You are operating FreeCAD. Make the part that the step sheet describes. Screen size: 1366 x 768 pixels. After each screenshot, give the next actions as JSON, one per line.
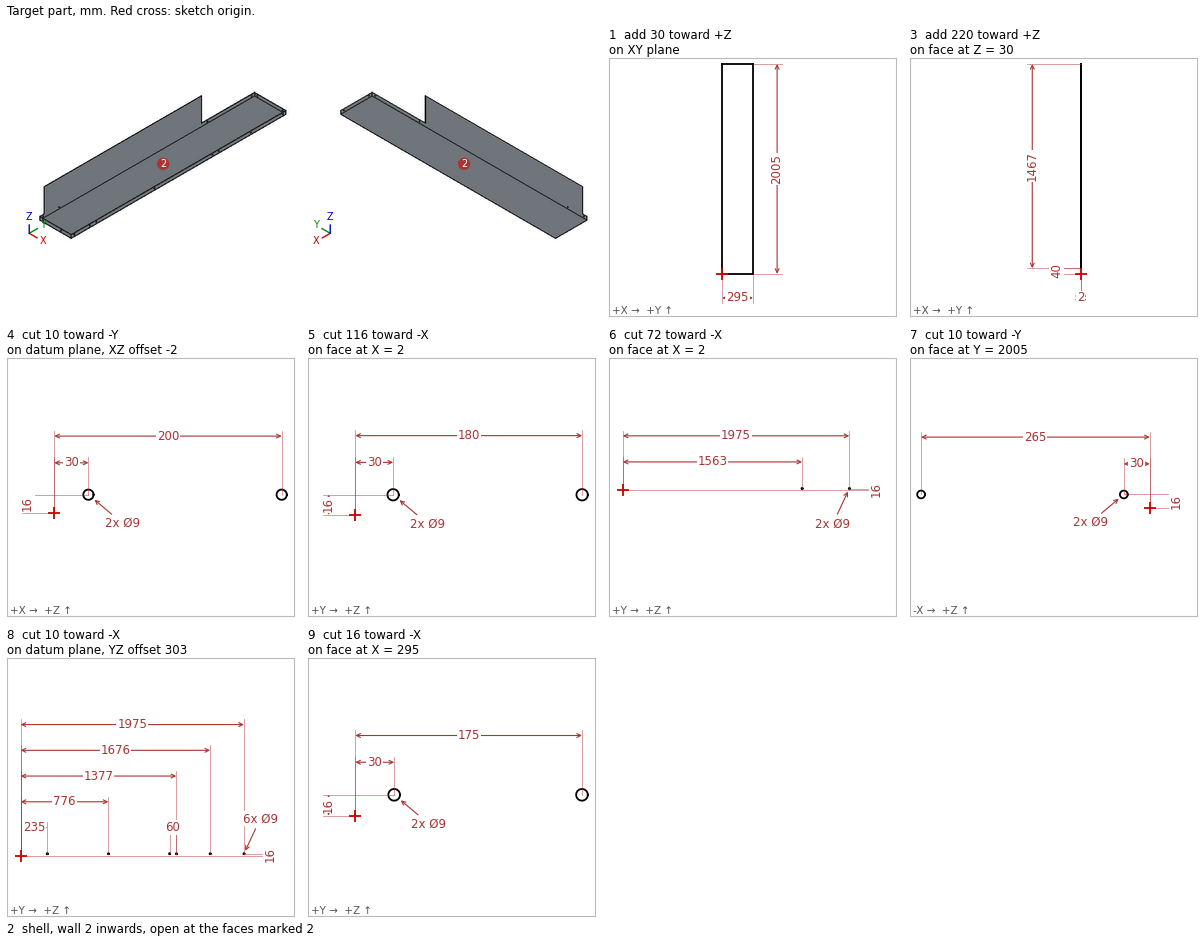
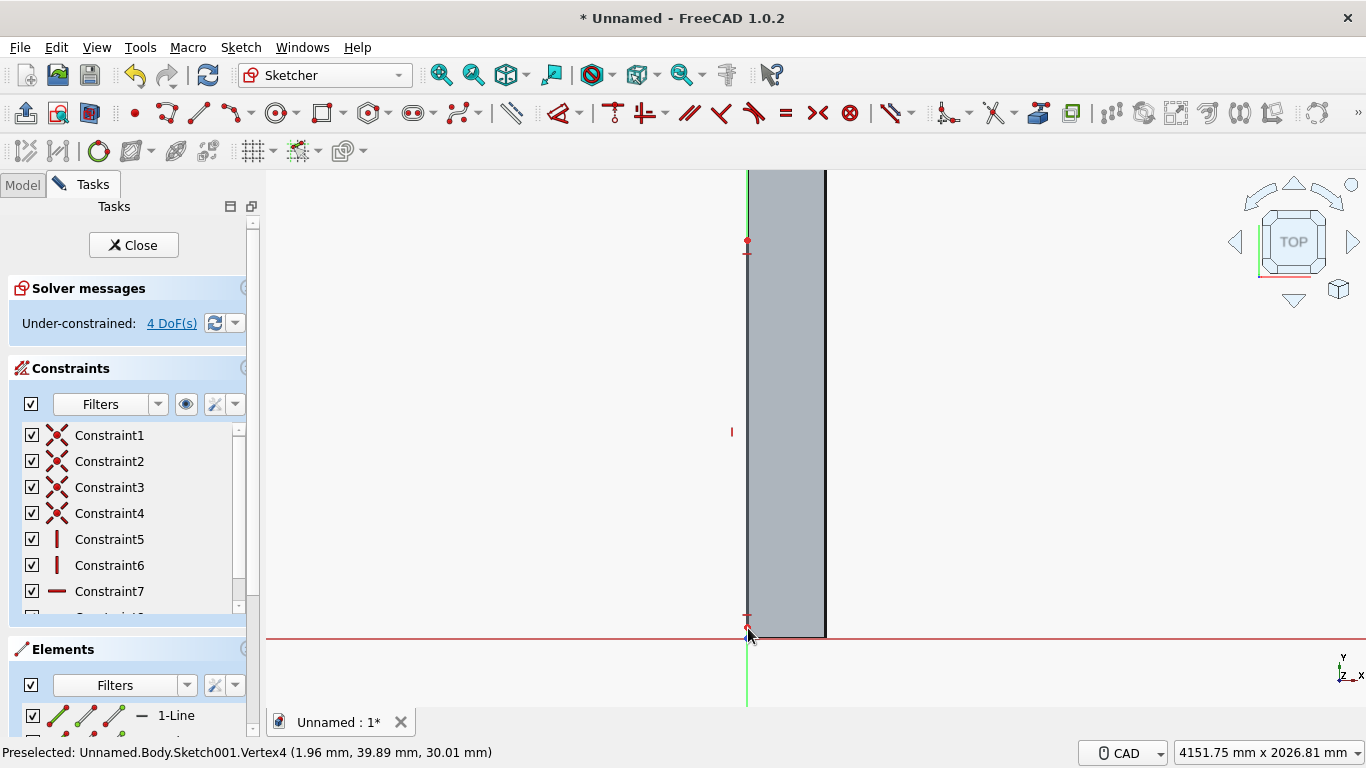
{"action": "scroll", "coordinate": [747, 240], "scroll_direction": "up", "scroll_amount": 13}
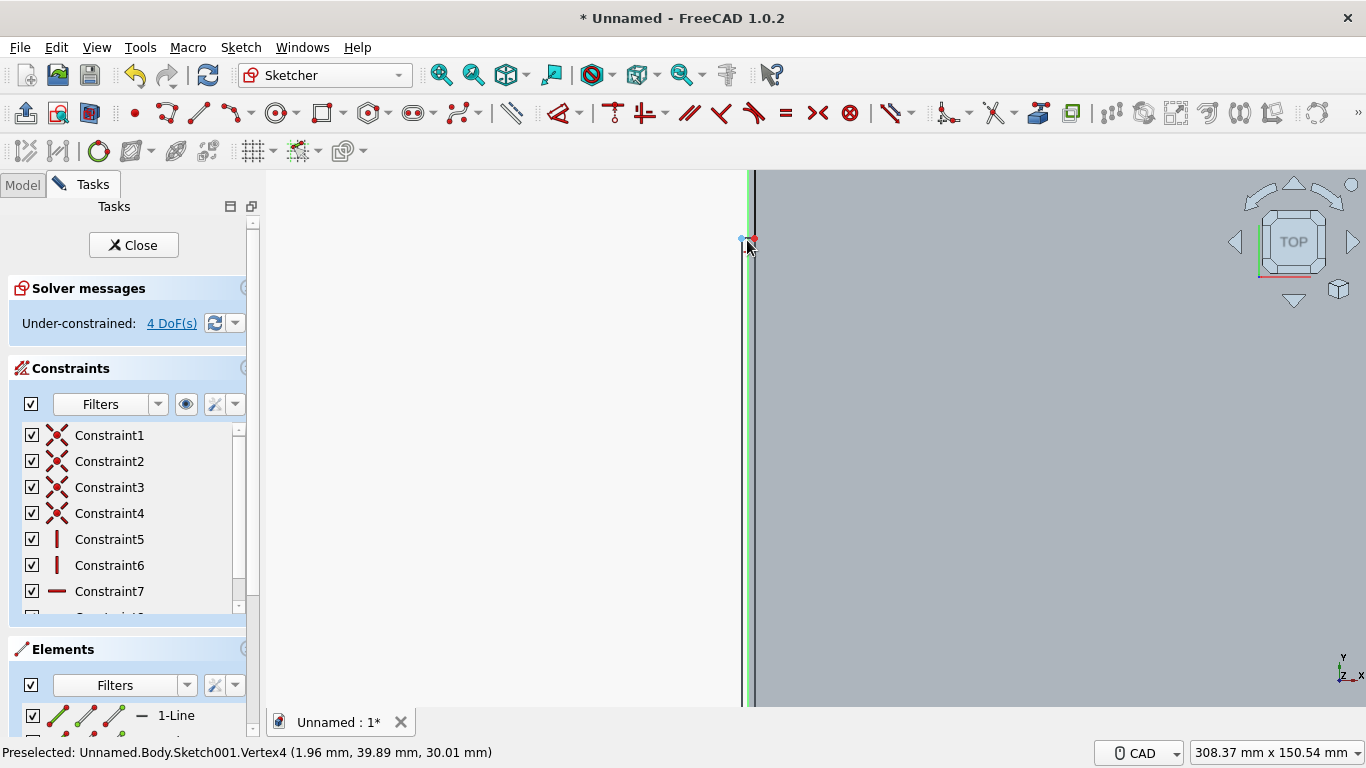
{"action": "left_click", "coordinate": [742, 238]}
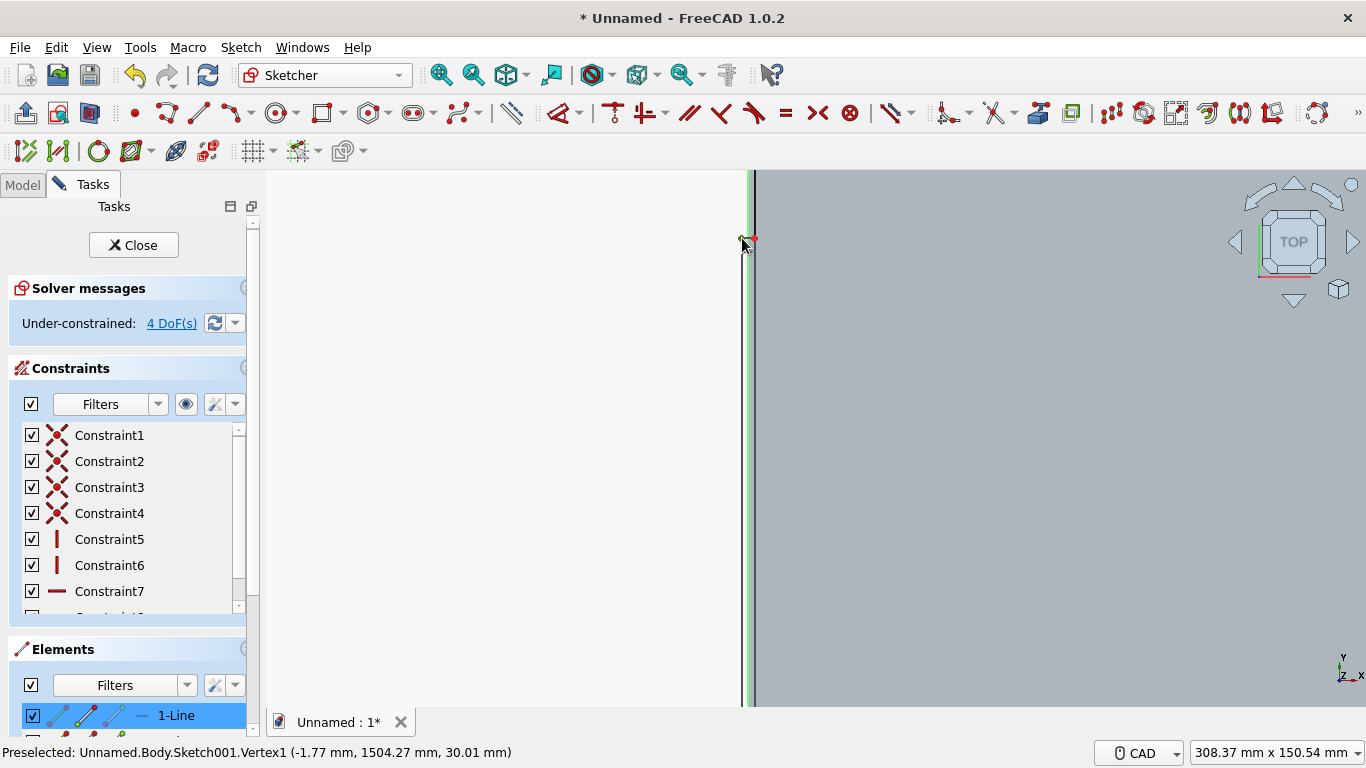
{"action": "left_click", "coordinate": [748, 645]}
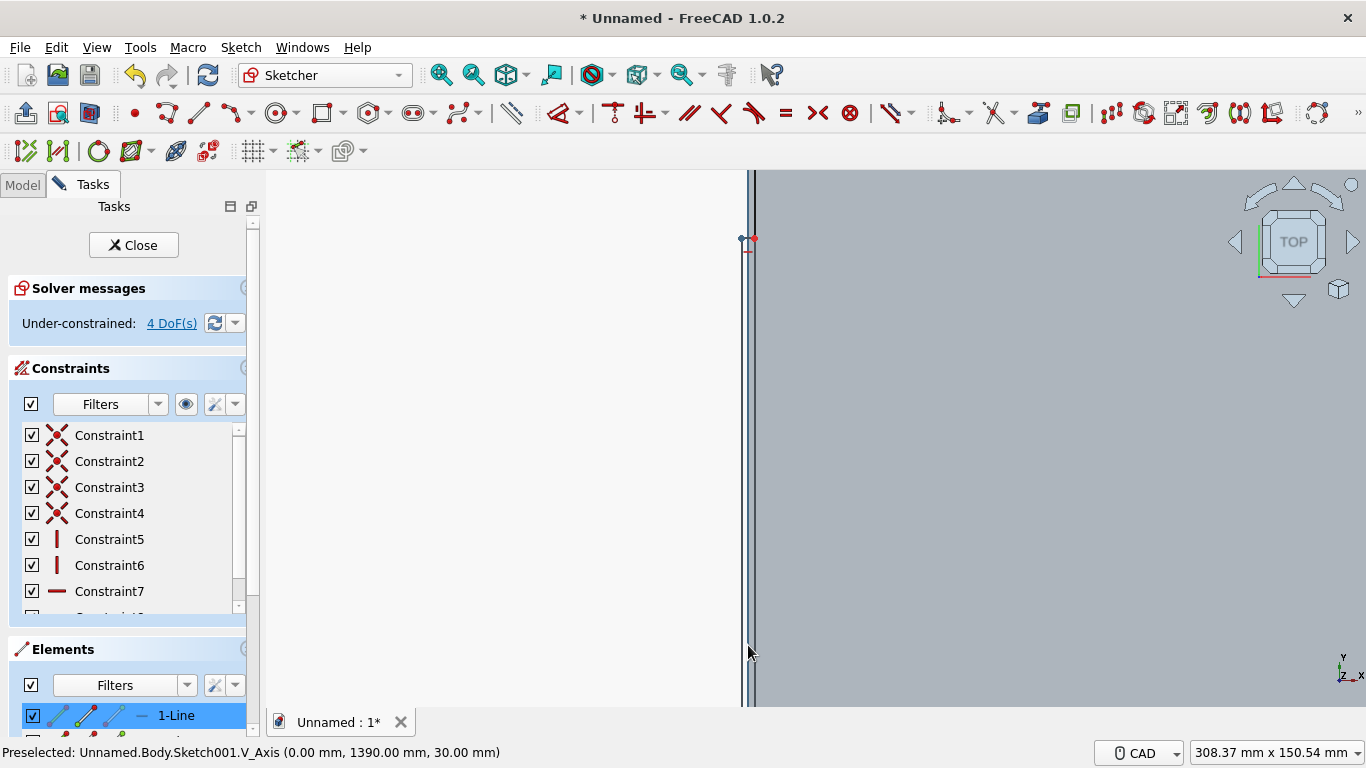
{"action": "left_click", "coordinate": [614, 114]}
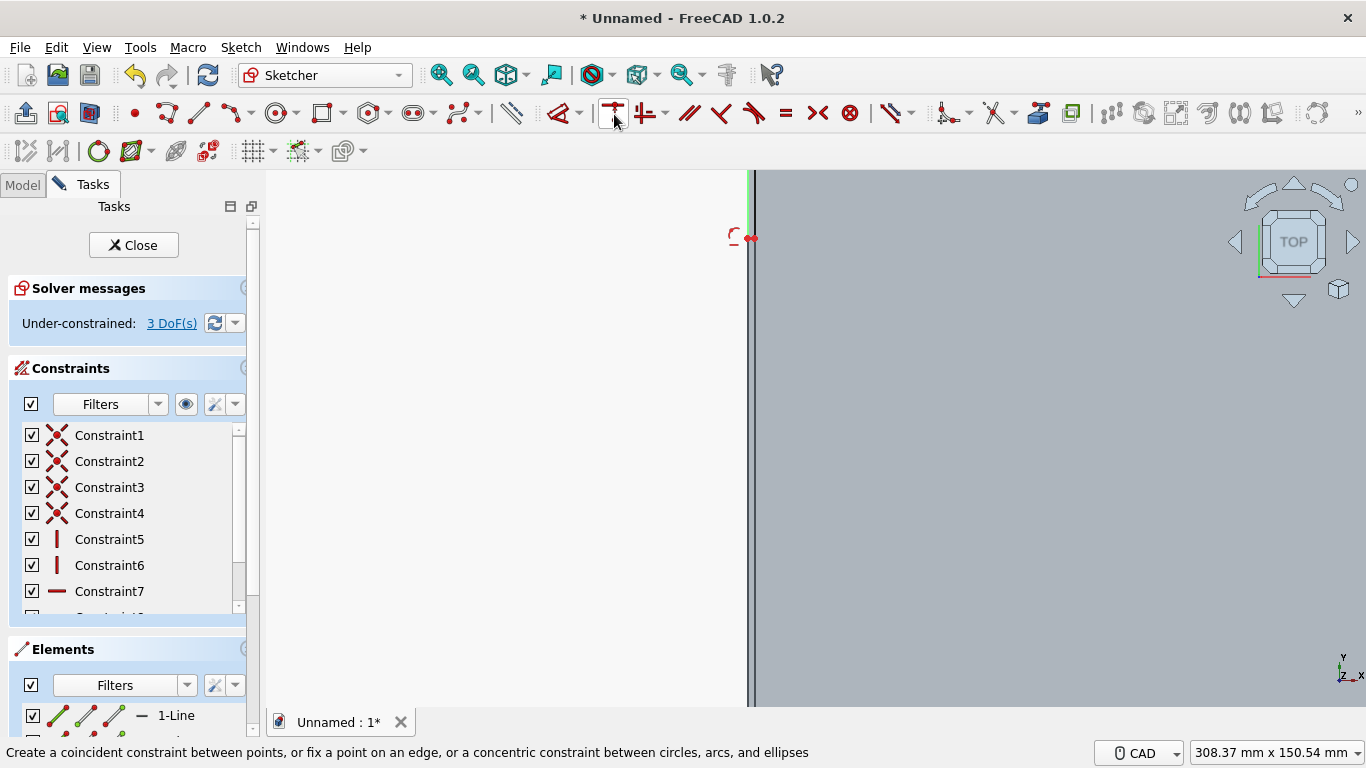
{"action": "left_click", "coordinate": [558, 114]}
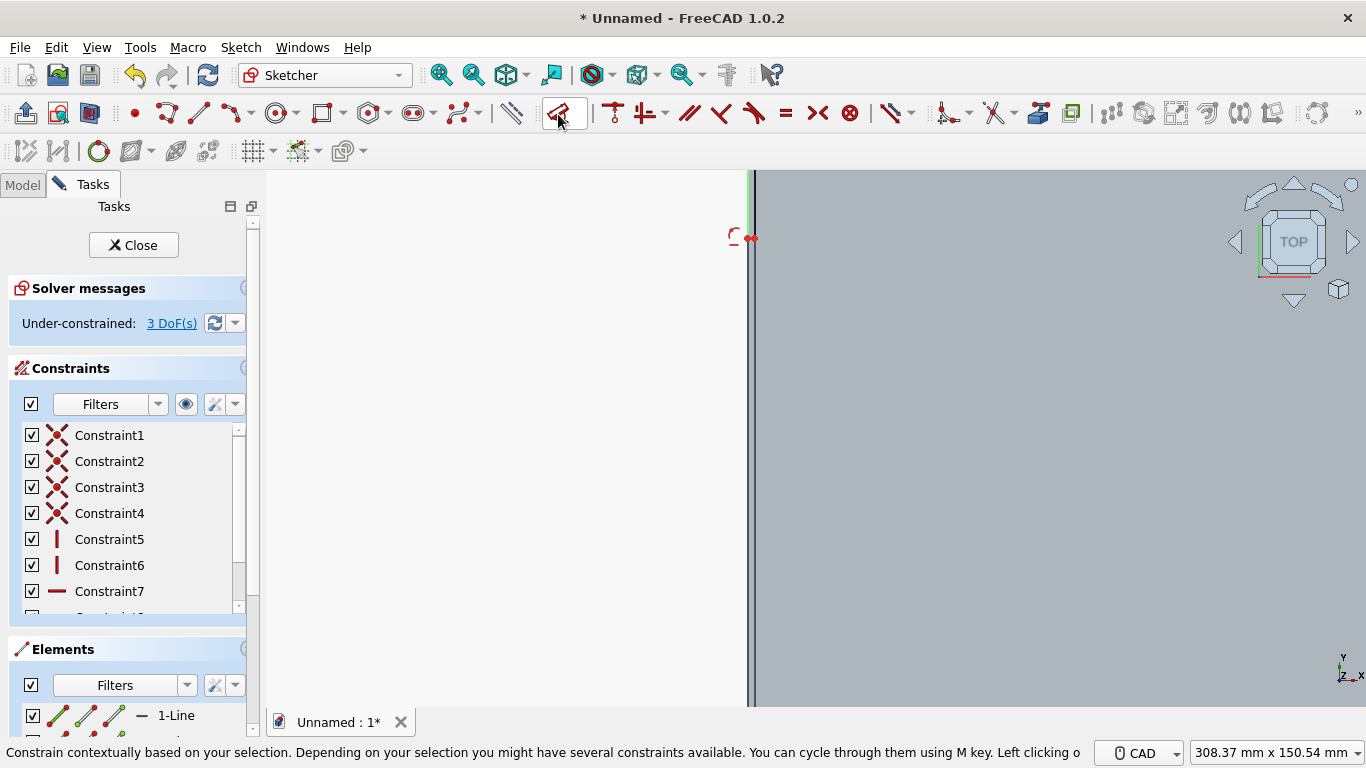
{"action": "scroll", "coordinate": [747, 278], "scroll_direction": "down", "scroll_amount": 14}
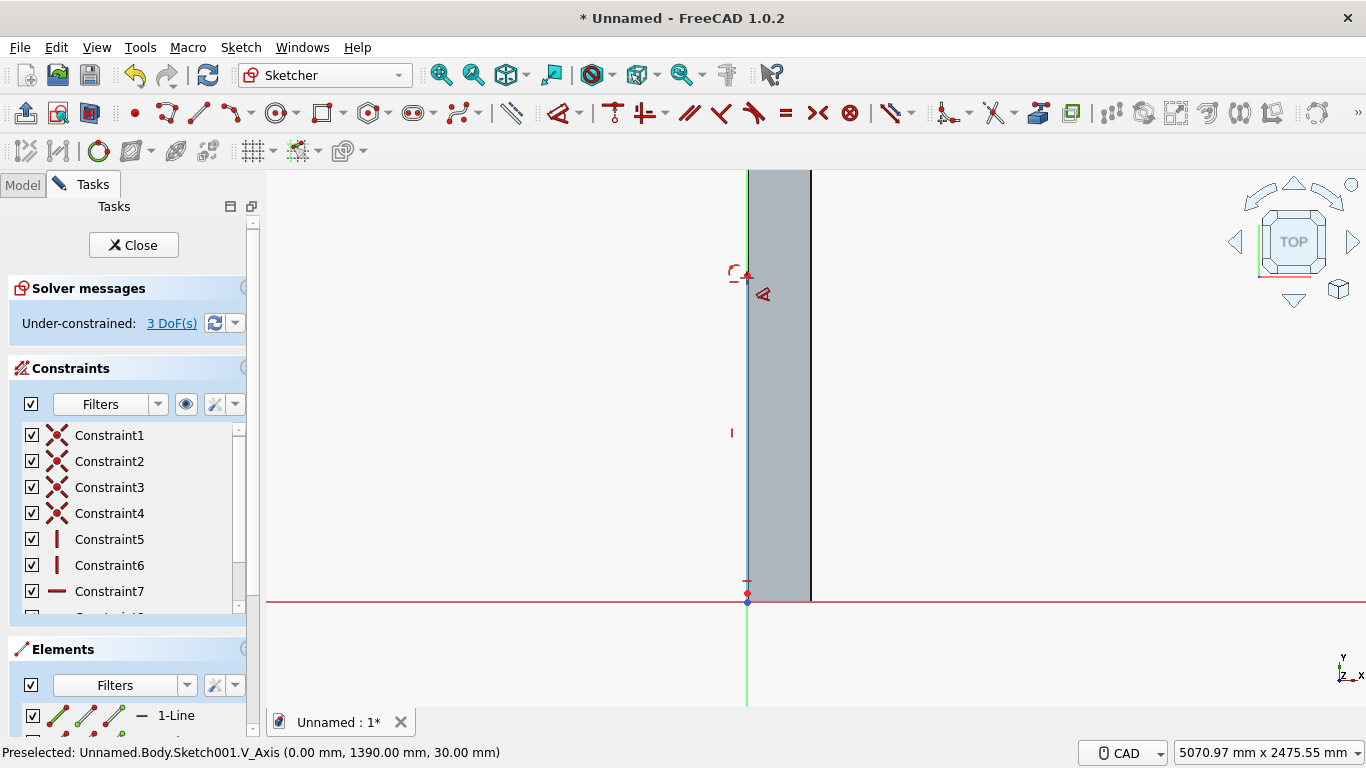
{"action": "scroll", "coordinate": [748, 593], "scroll_direction": "up", "scroll_amount": 23}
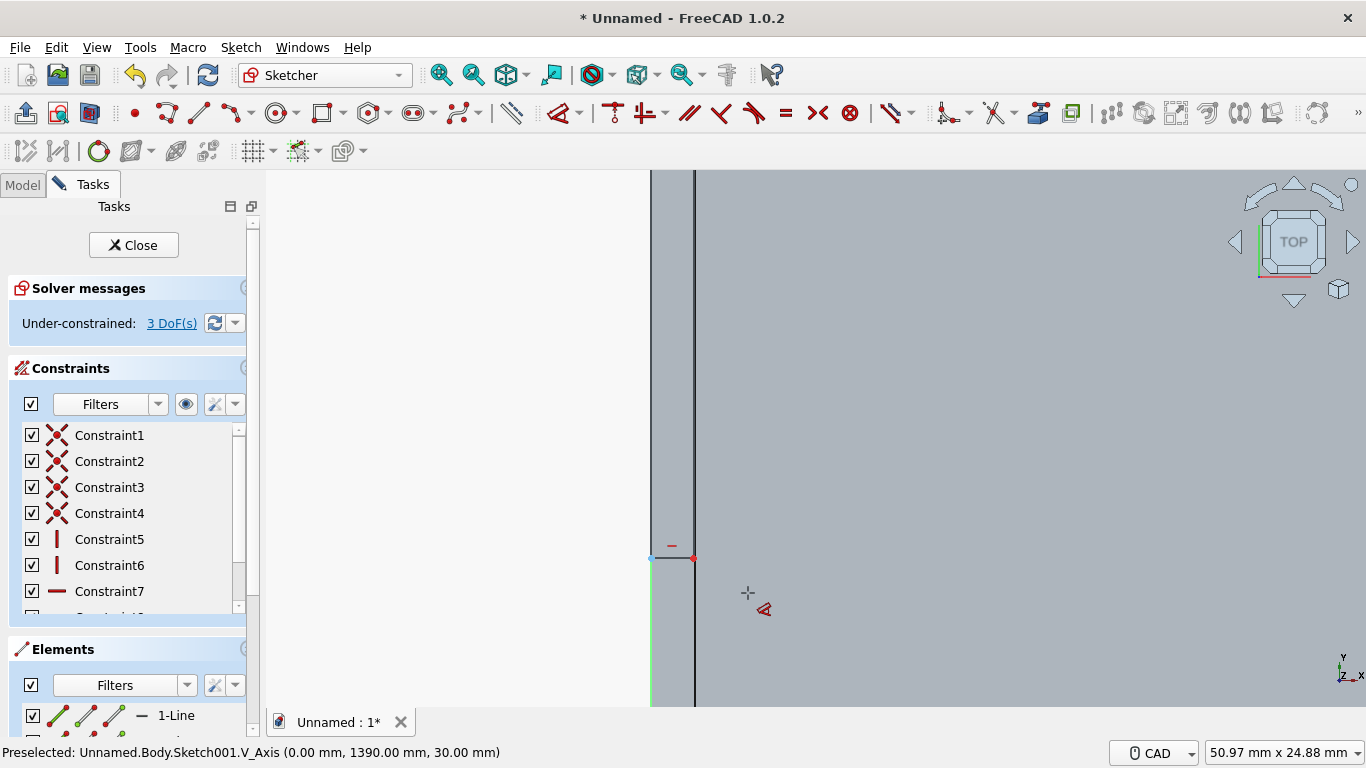
{"action": "left_click", "coordinate": [673, 558]}
{"action": "left_click", "coordinate": [673, 592]}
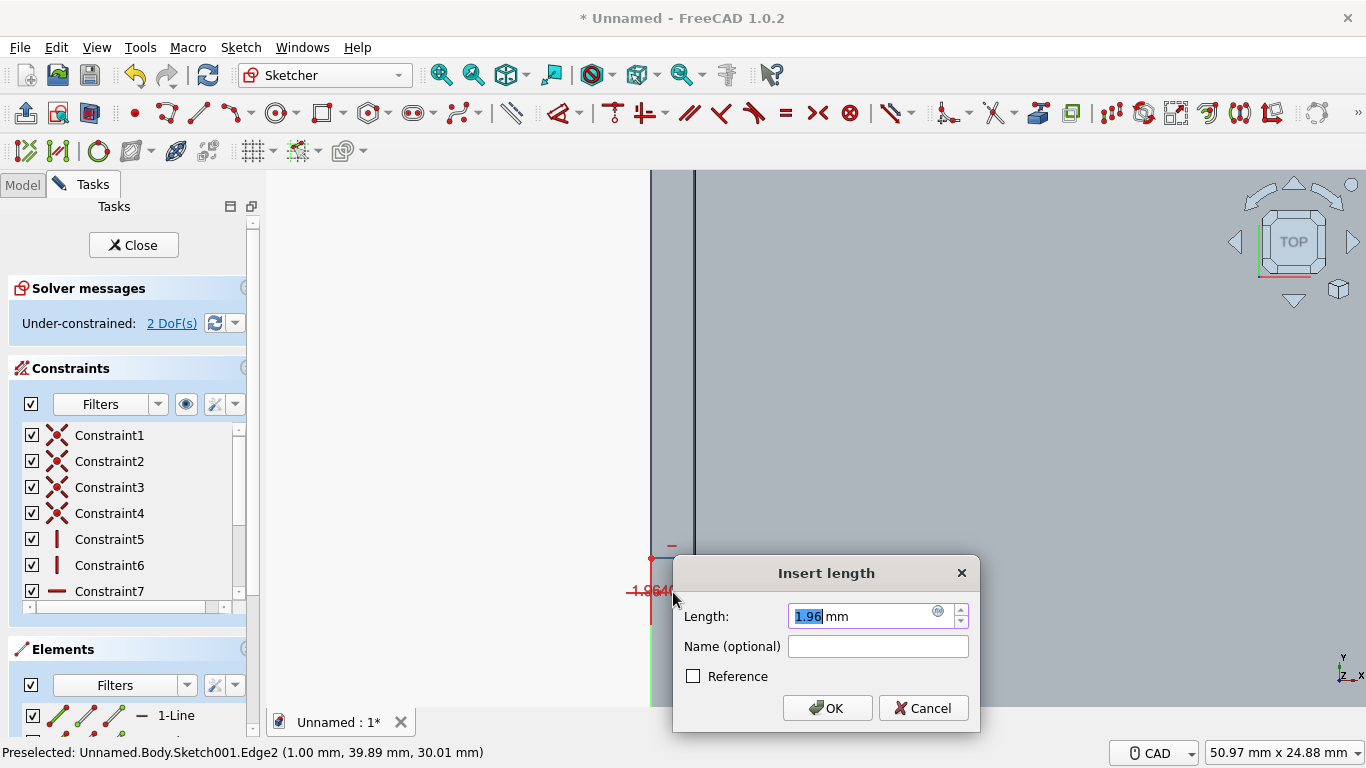
{"action": "type", "text": "2"}
{"action": "key", "text": "Return"}